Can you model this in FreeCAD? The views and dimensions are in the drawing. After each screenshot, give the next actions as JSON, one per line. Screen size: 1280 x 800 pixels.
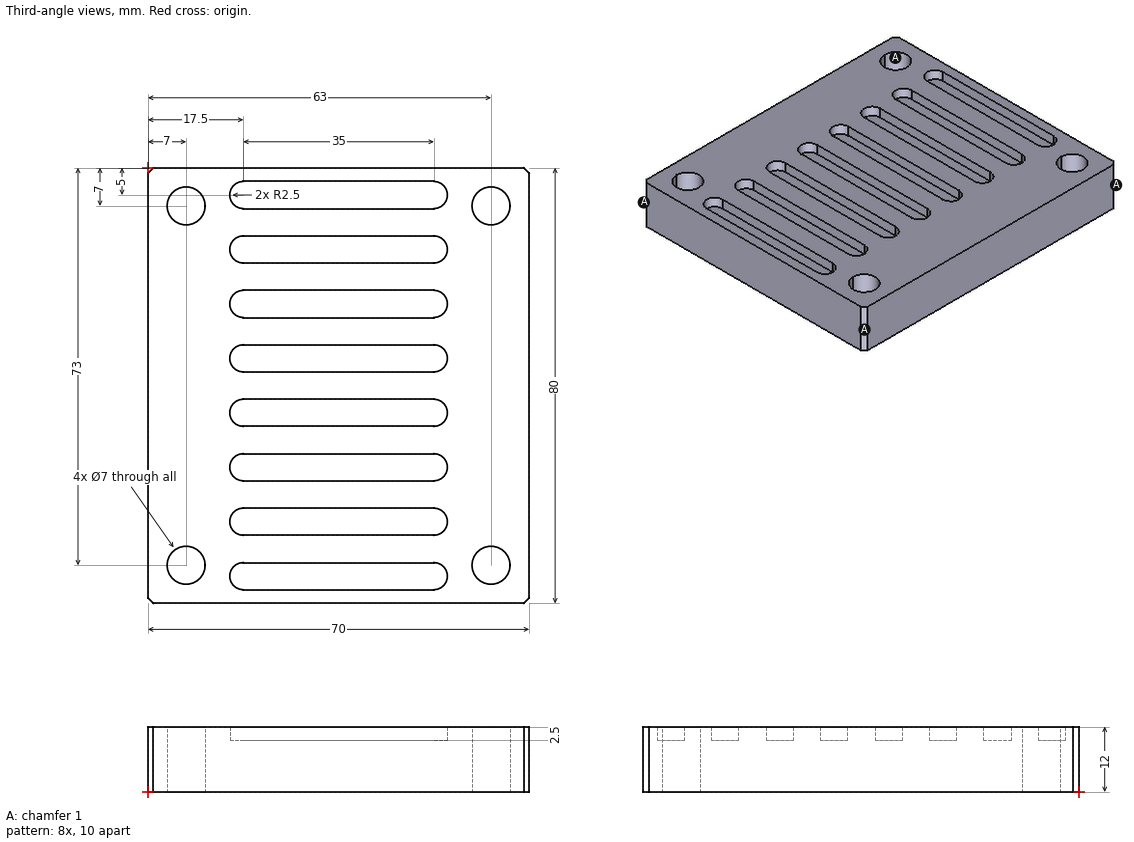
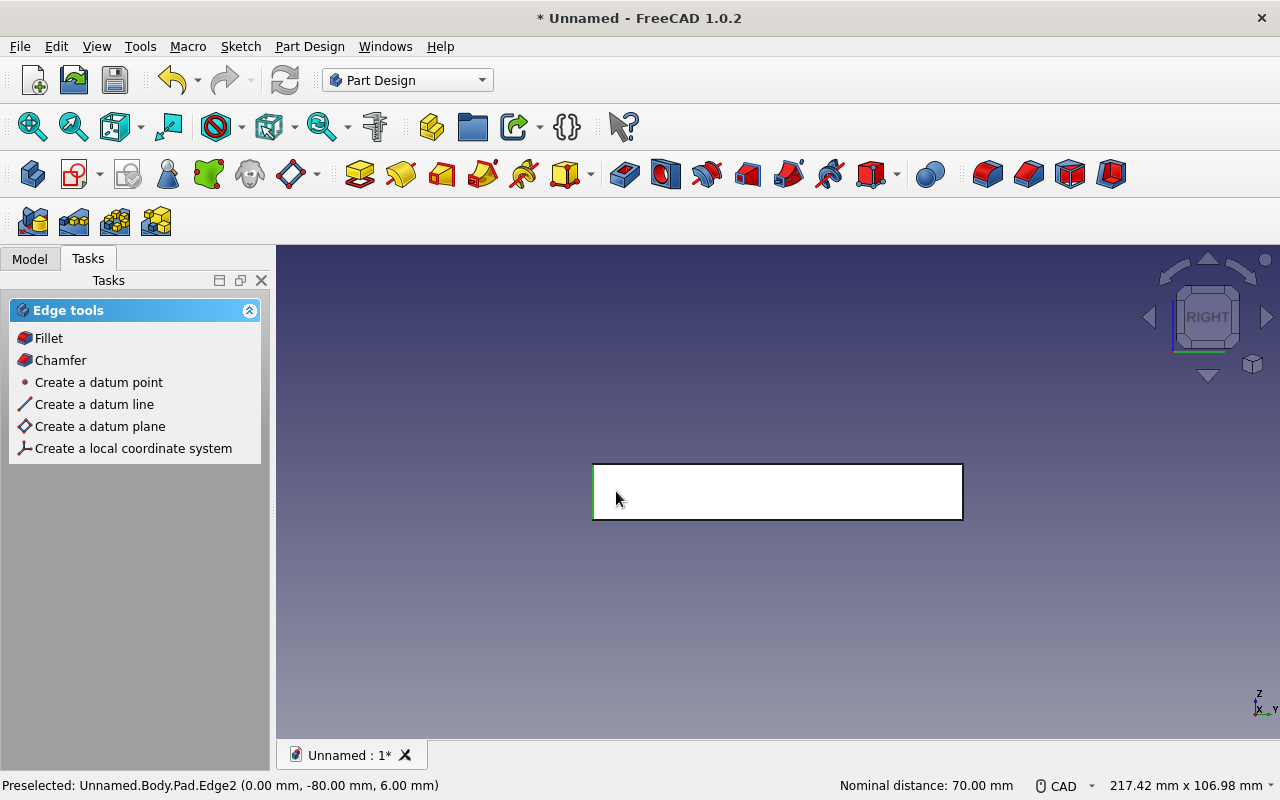
{"action": "key", "text": "v f"}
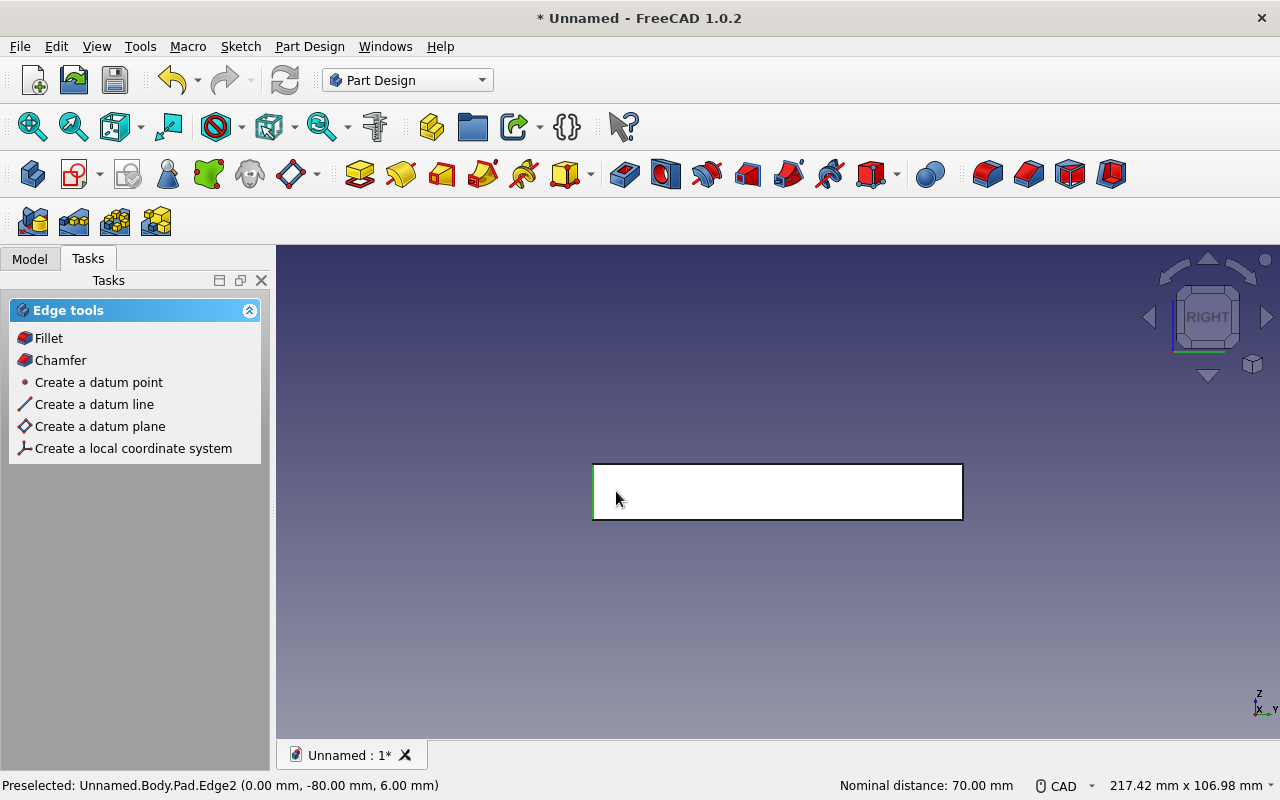
{"action": "left_click", "coordinate": [963, 491], "text": "ctrl"}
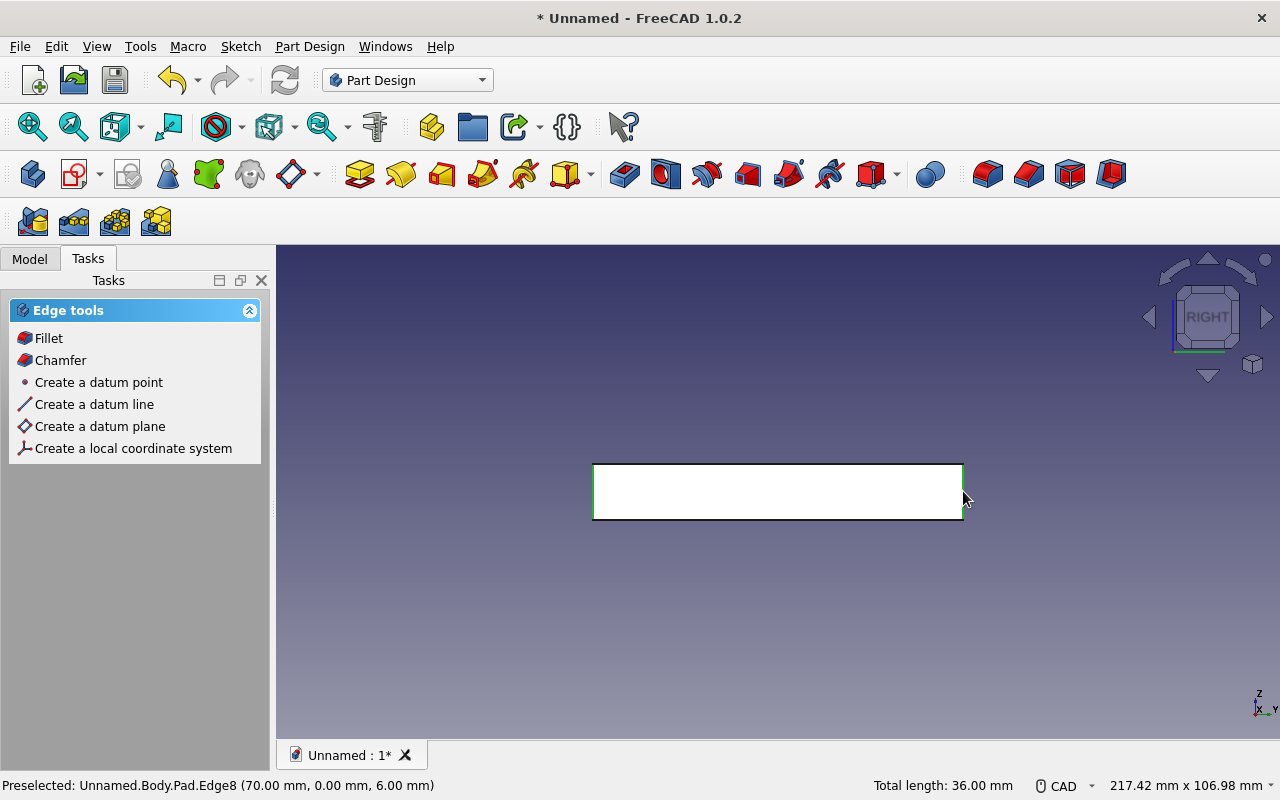
{"action": "key", "text": "5"}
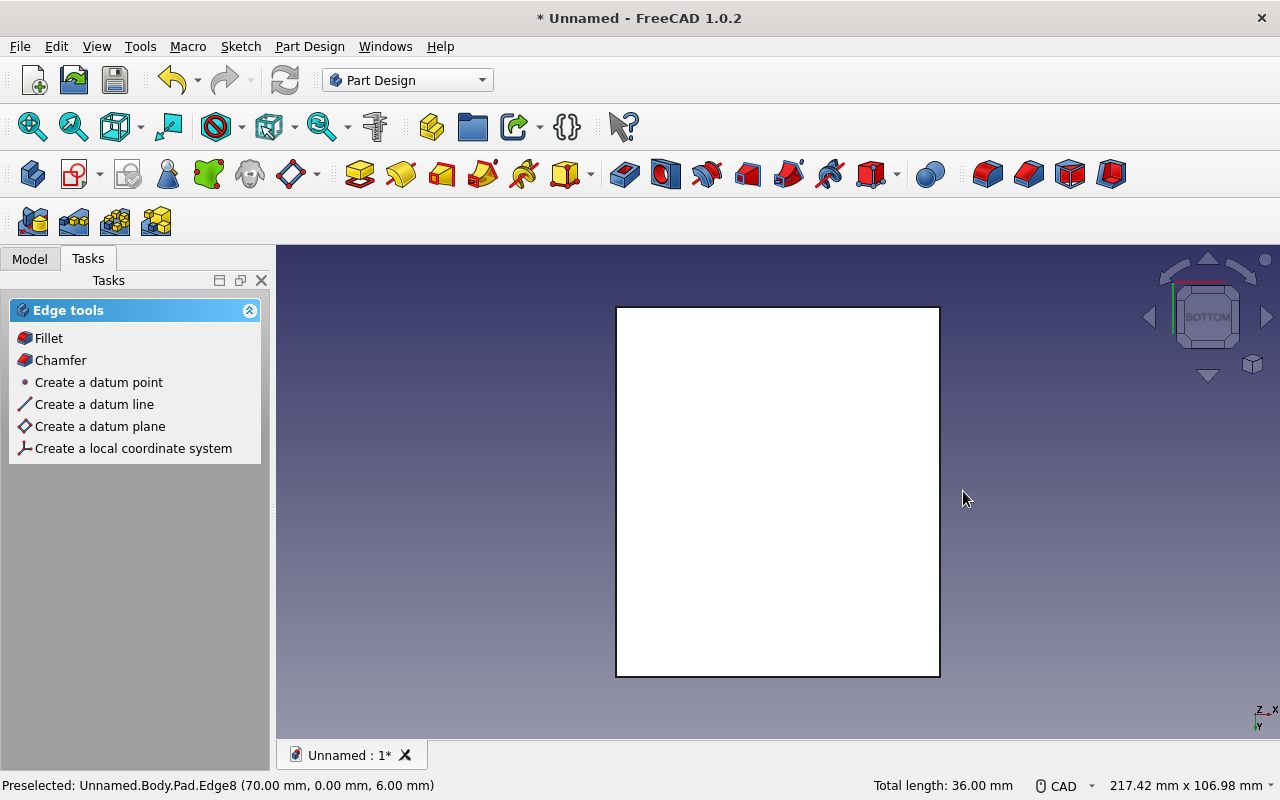
{"action": "key", "text": "4"}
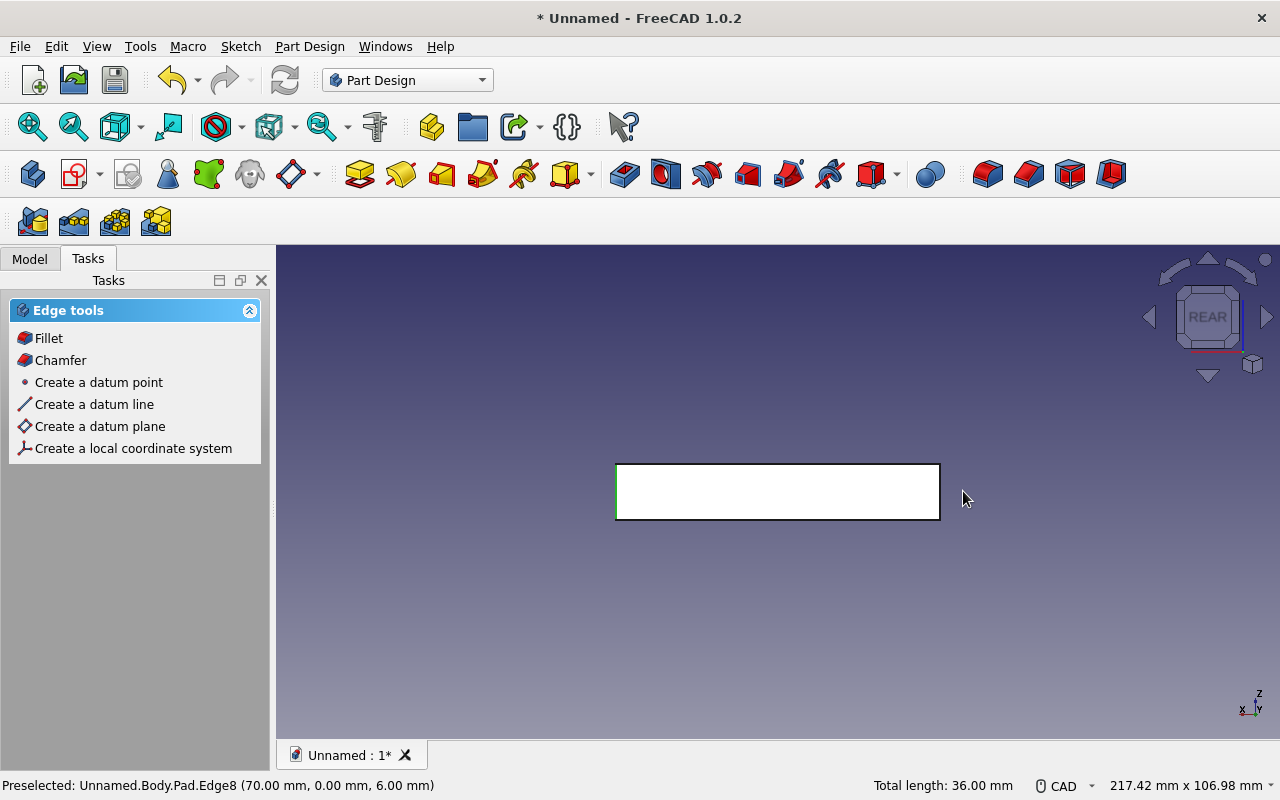
{"action": "key", "text": "v f"}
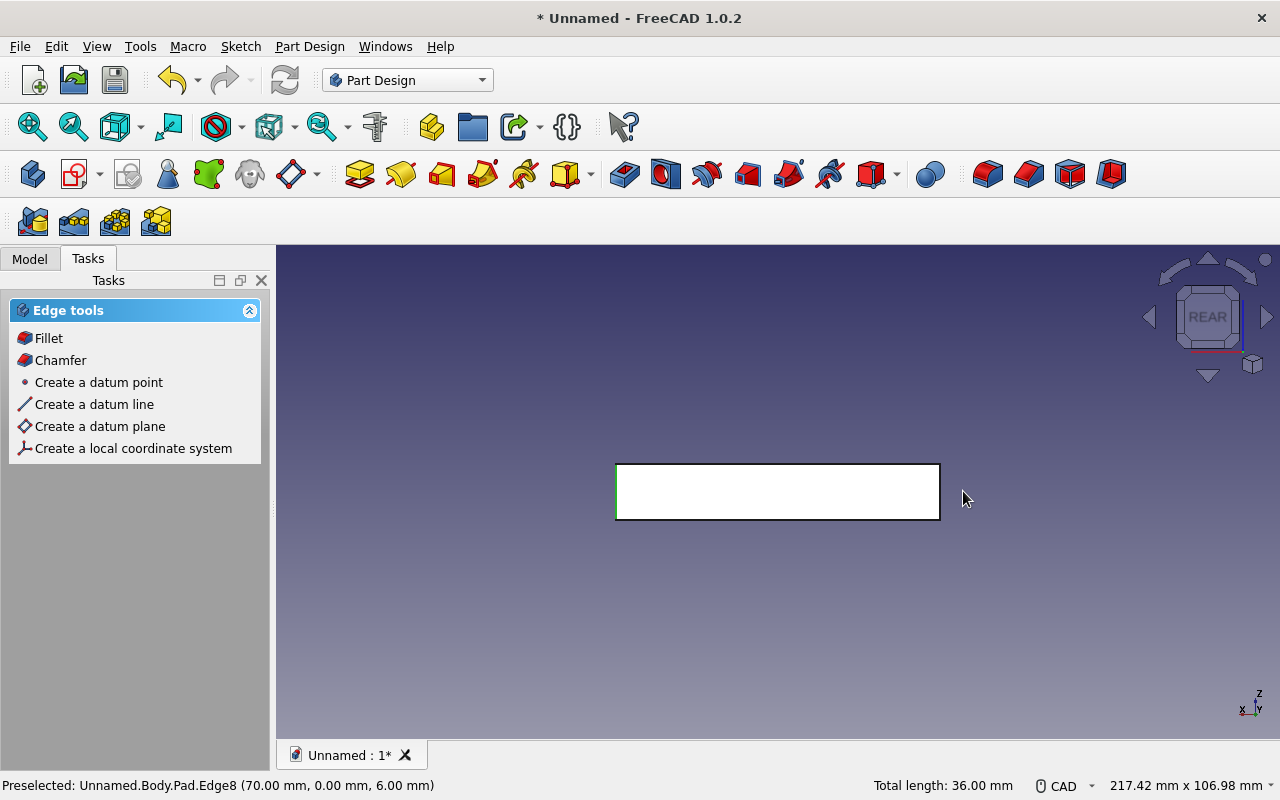
{"action": "left_click", "coordinate": [940, 491], "text": "ctrl"}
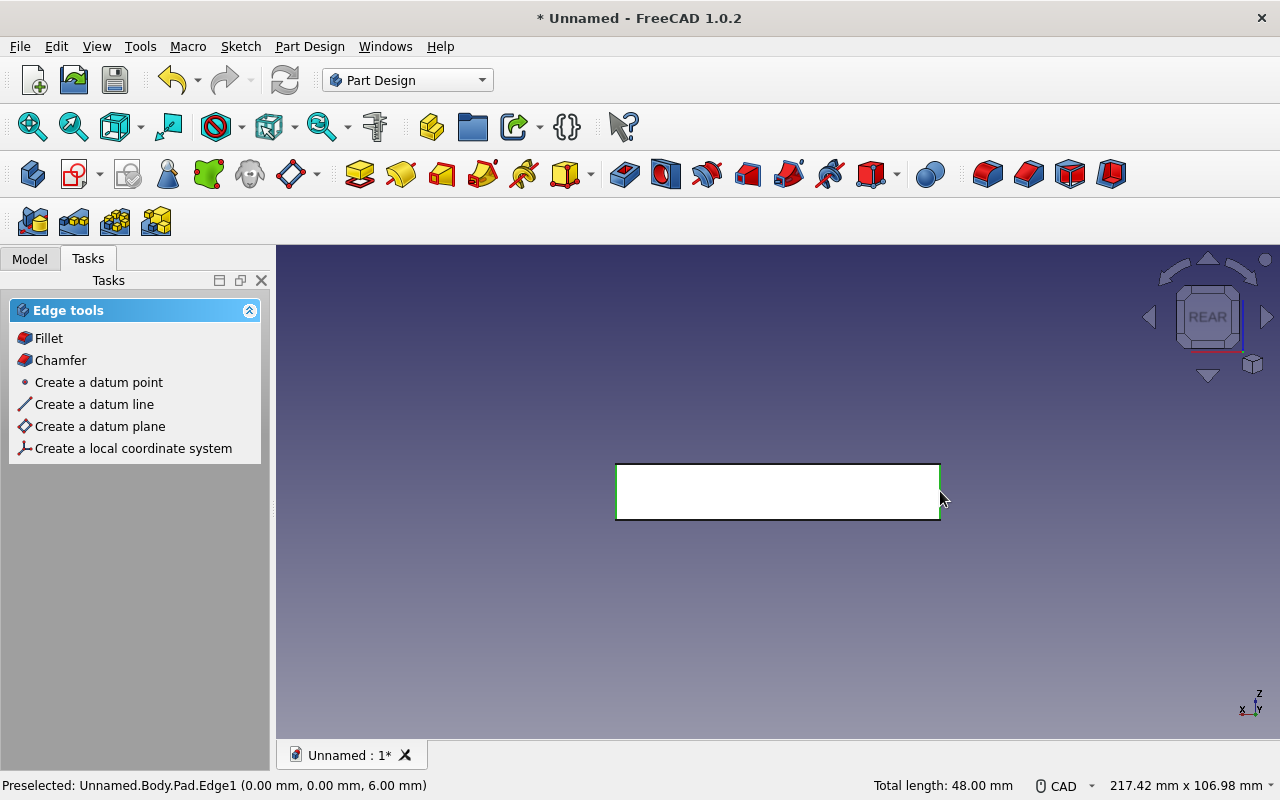
{"action": "left_click", "coordinate": [1029, 174]}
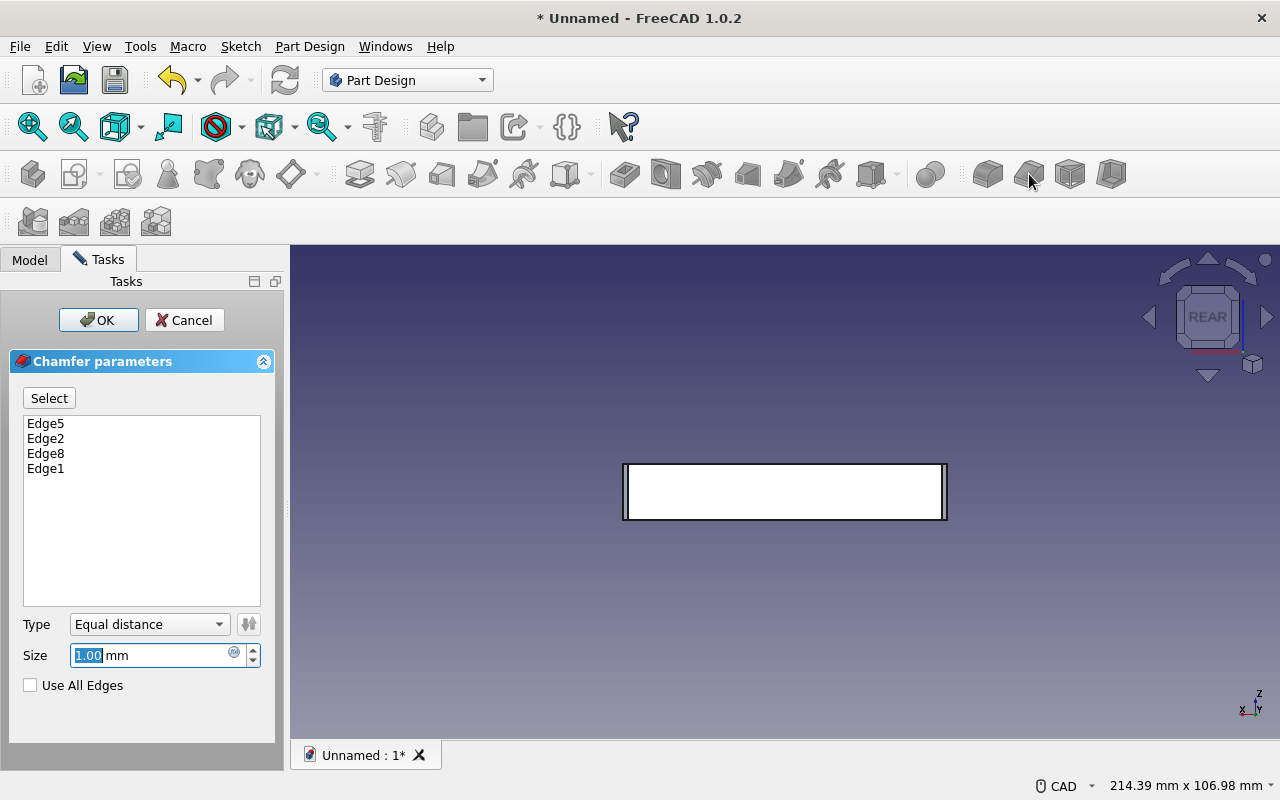
{"action": "type", "text": "1"}
{"action": "key", "text": "Tab"}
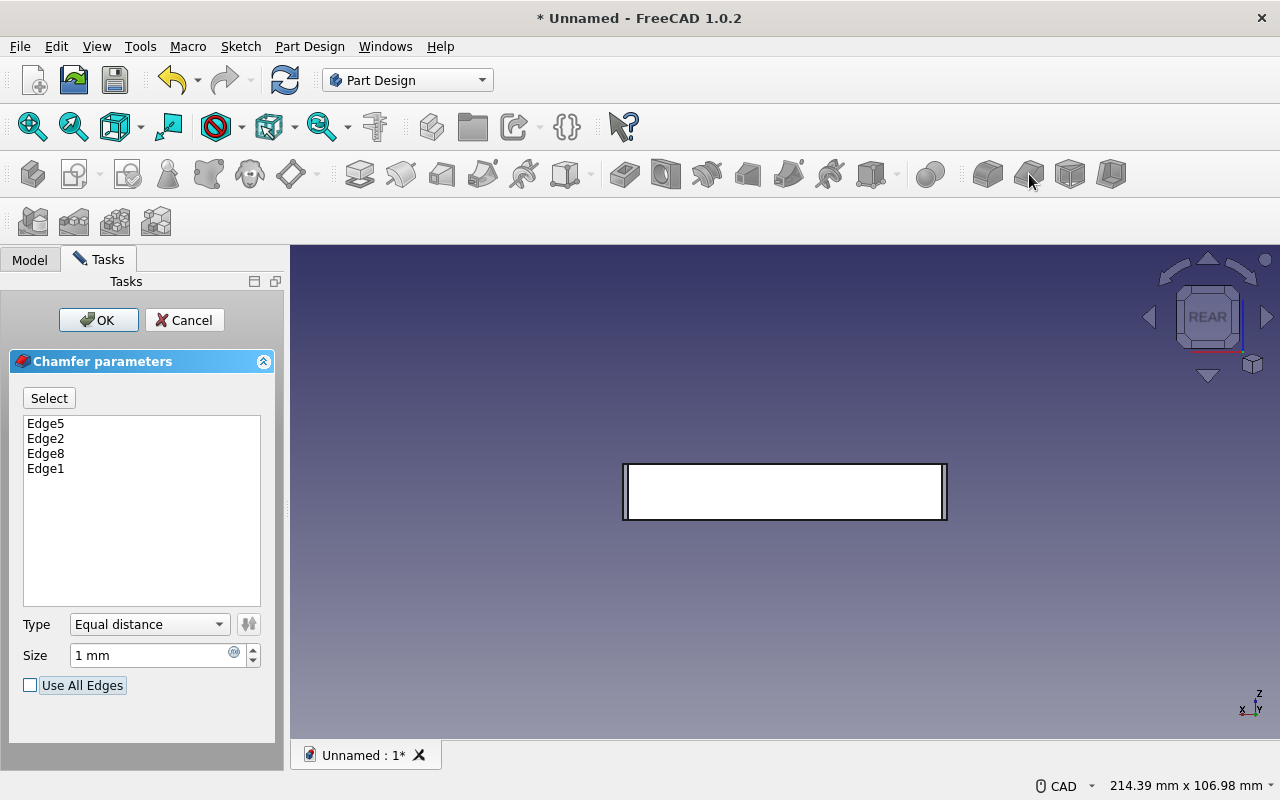
{"action": "left_click", "coordinate": [99, 320]}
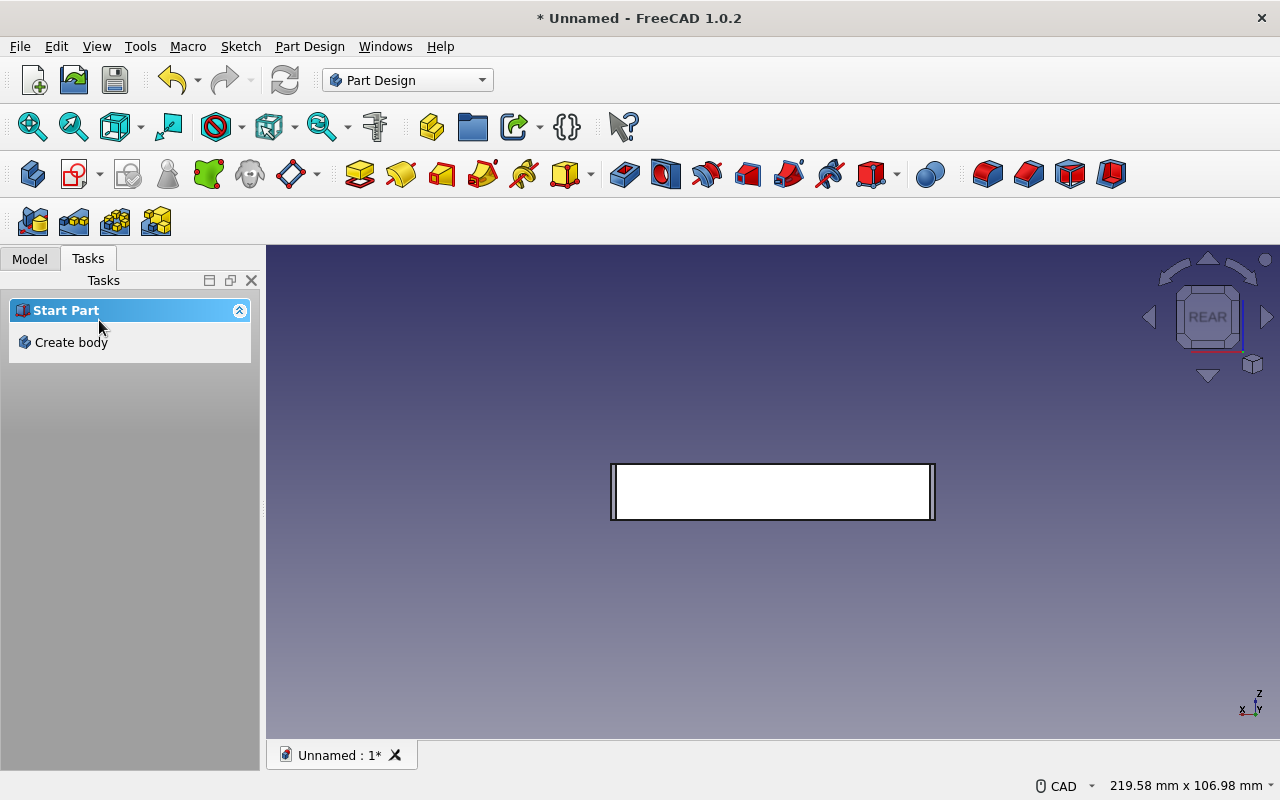
{"action": "key", "text": "v f"}